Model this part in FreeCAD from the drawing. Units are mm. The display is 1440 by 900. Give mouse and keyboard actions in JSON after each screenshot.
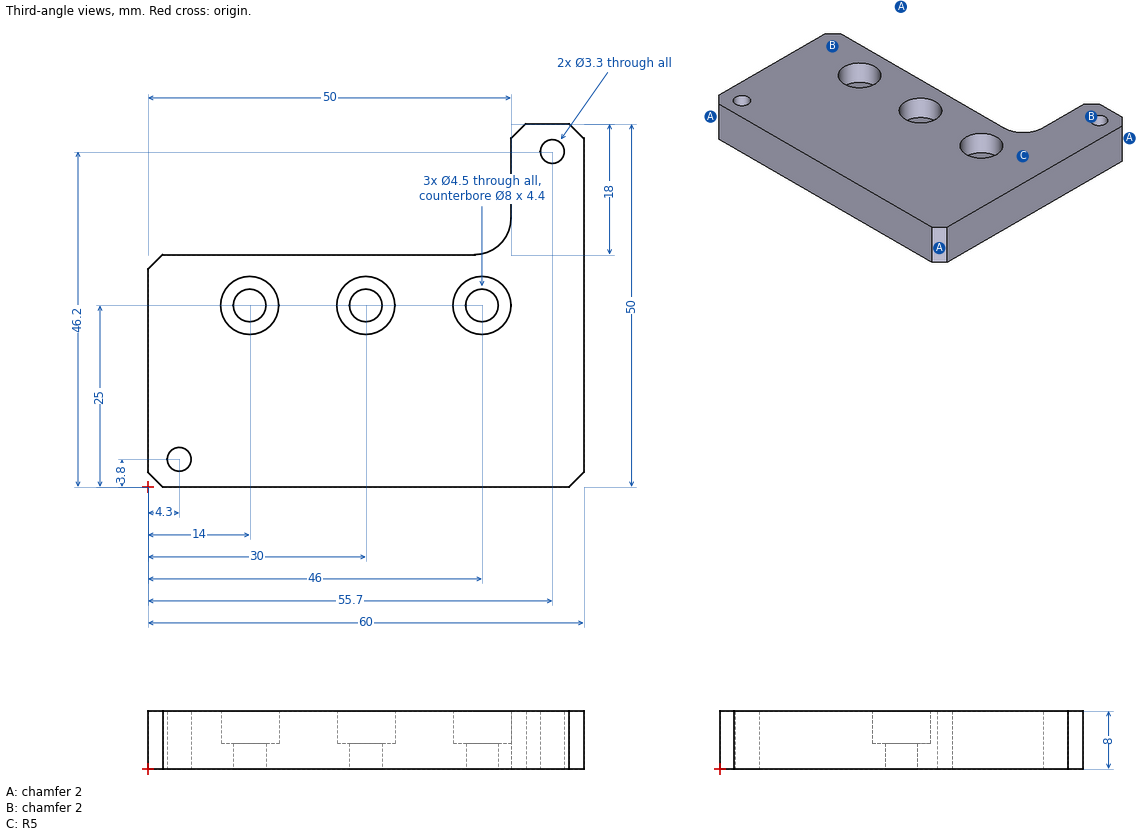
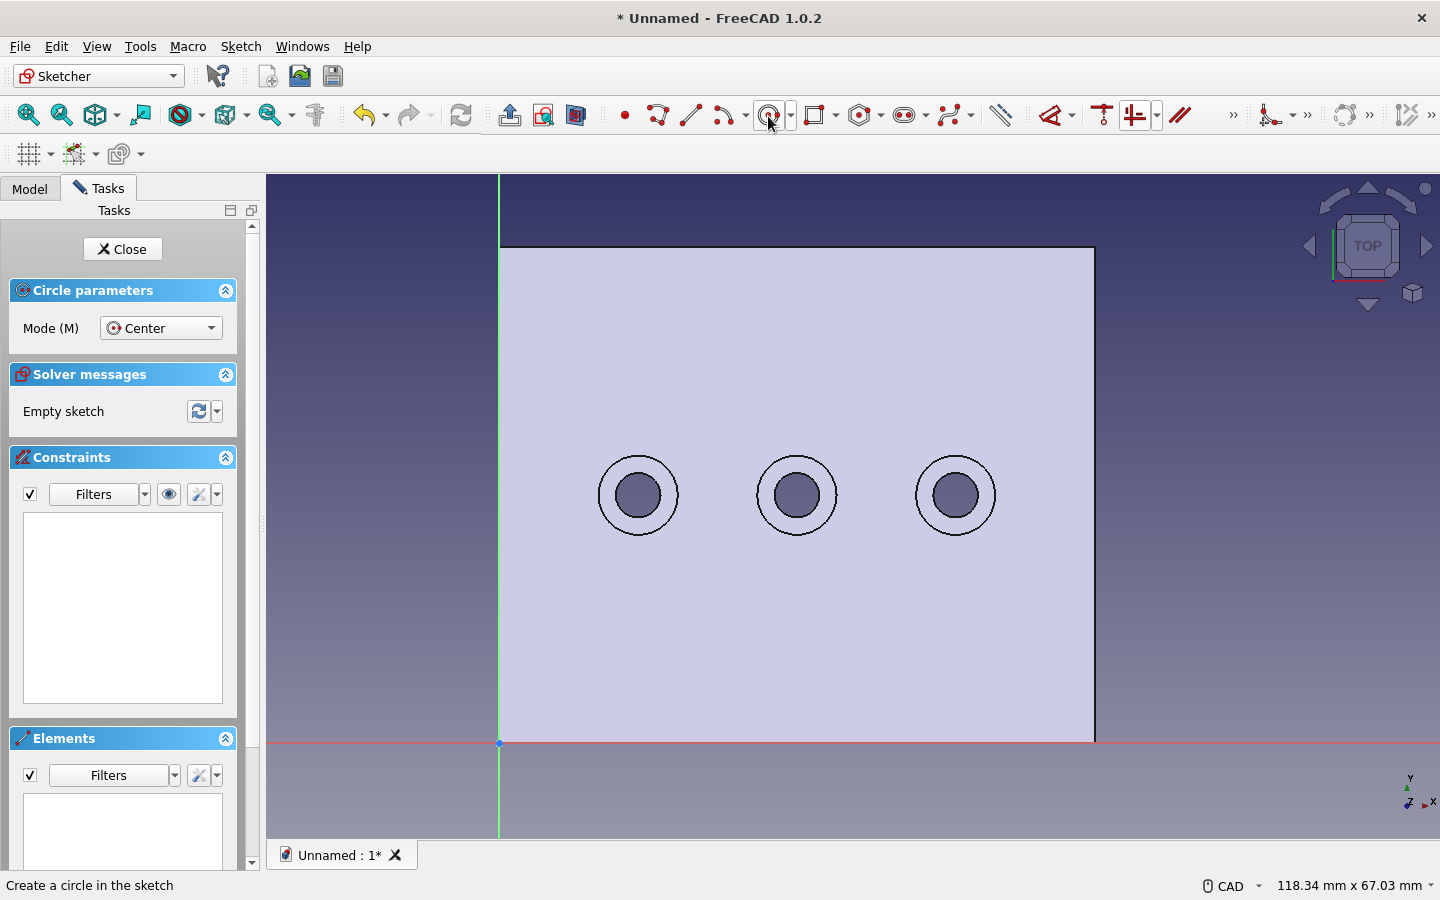
{"action": "scroll", "coordinate": [1052, 285], "scroll_direction": "up", "scroll_amount": 2}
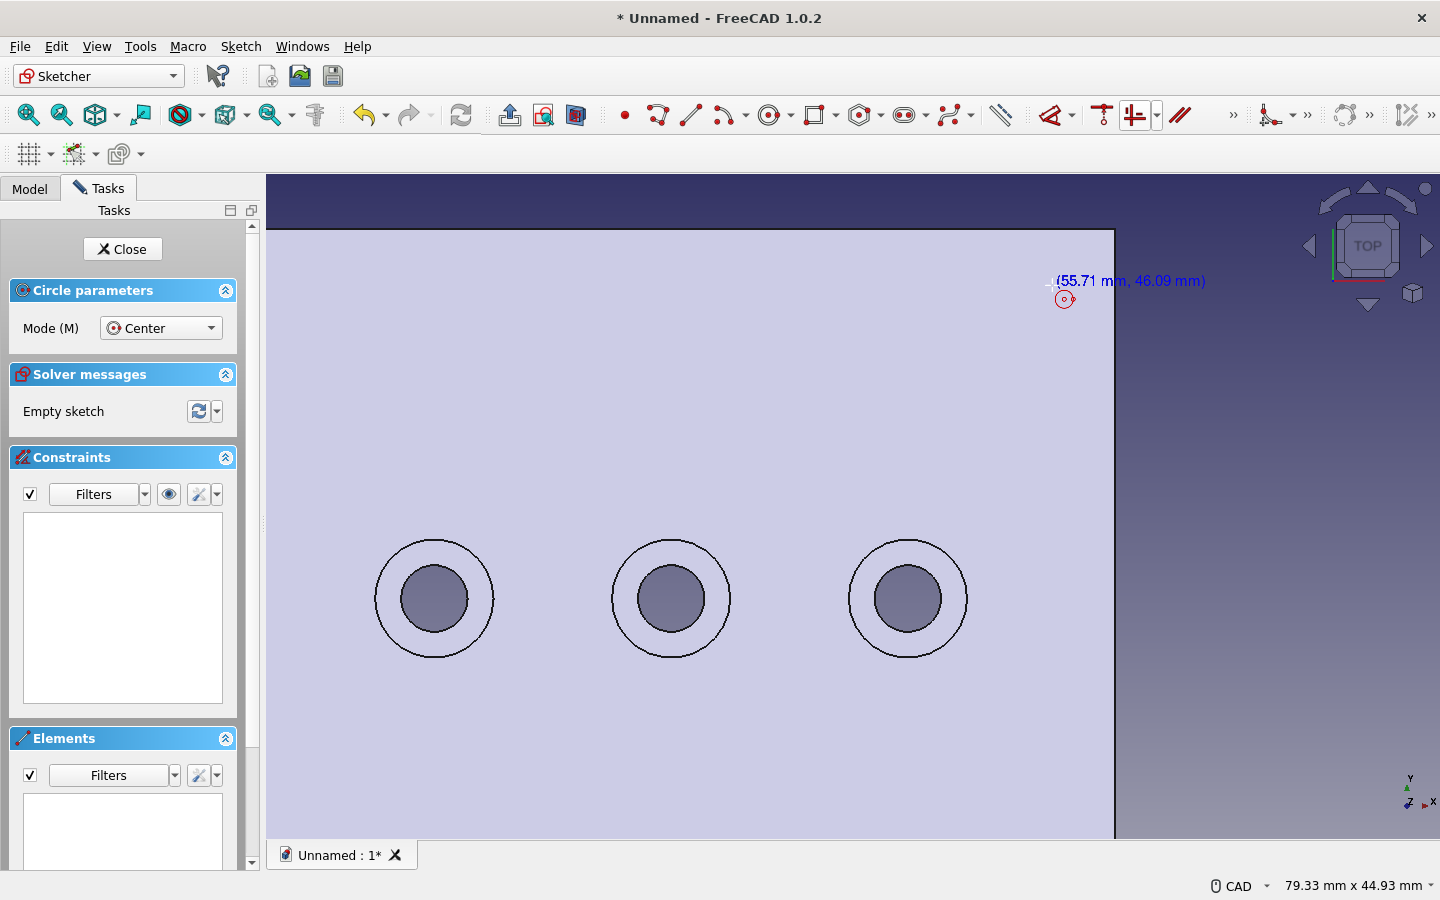
{"action": "left_click", "coordinate": [1051, 285]}
{"action": "mouse_move", "coordinate": [1069, 268]}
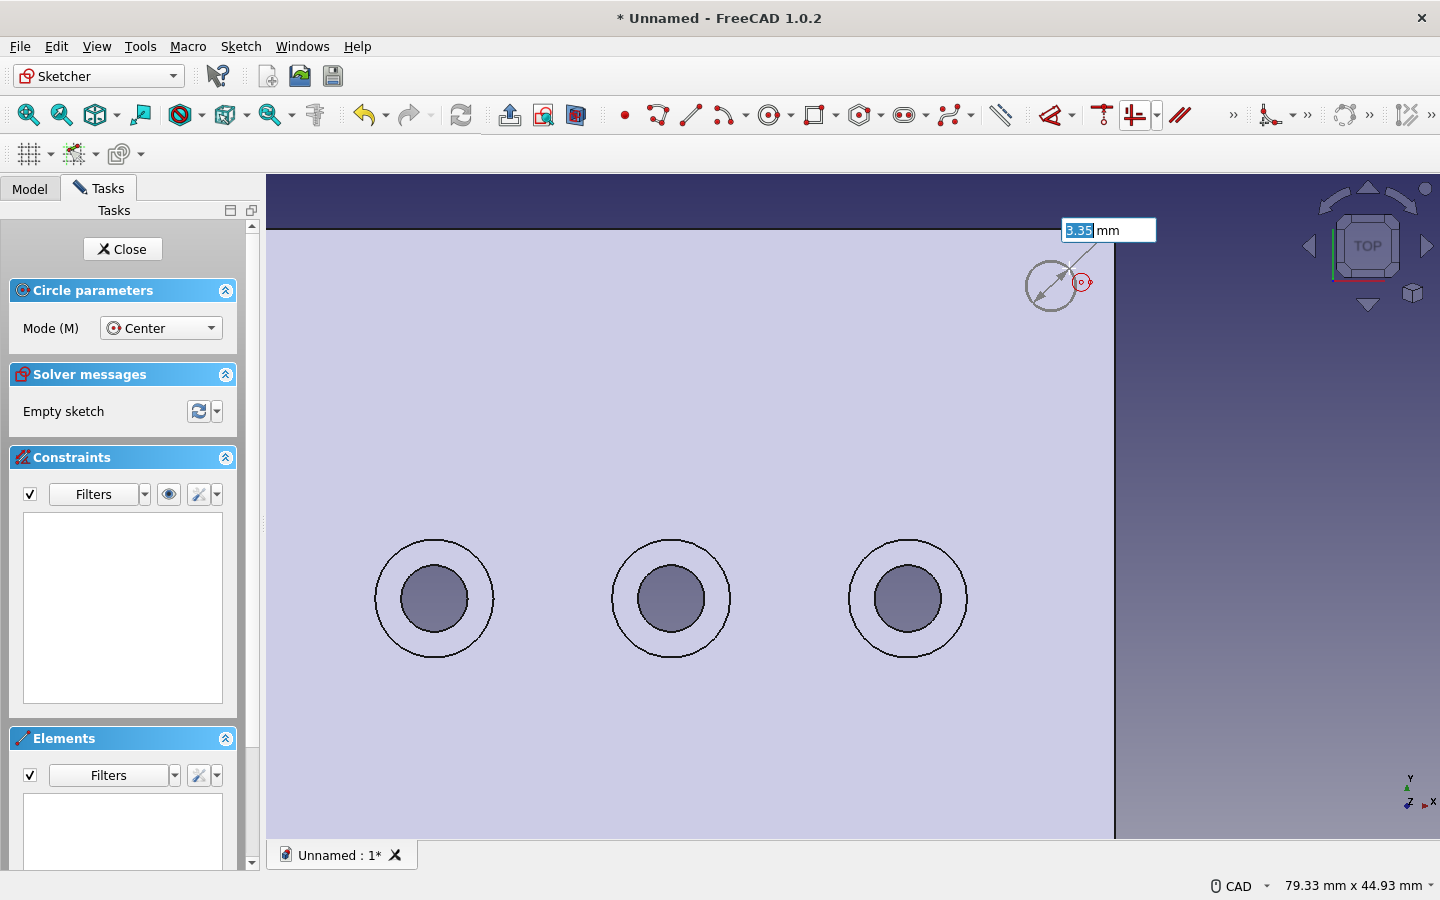
{"action": "type", "text": "3.3"}
{"action": "key", "text": "Return"}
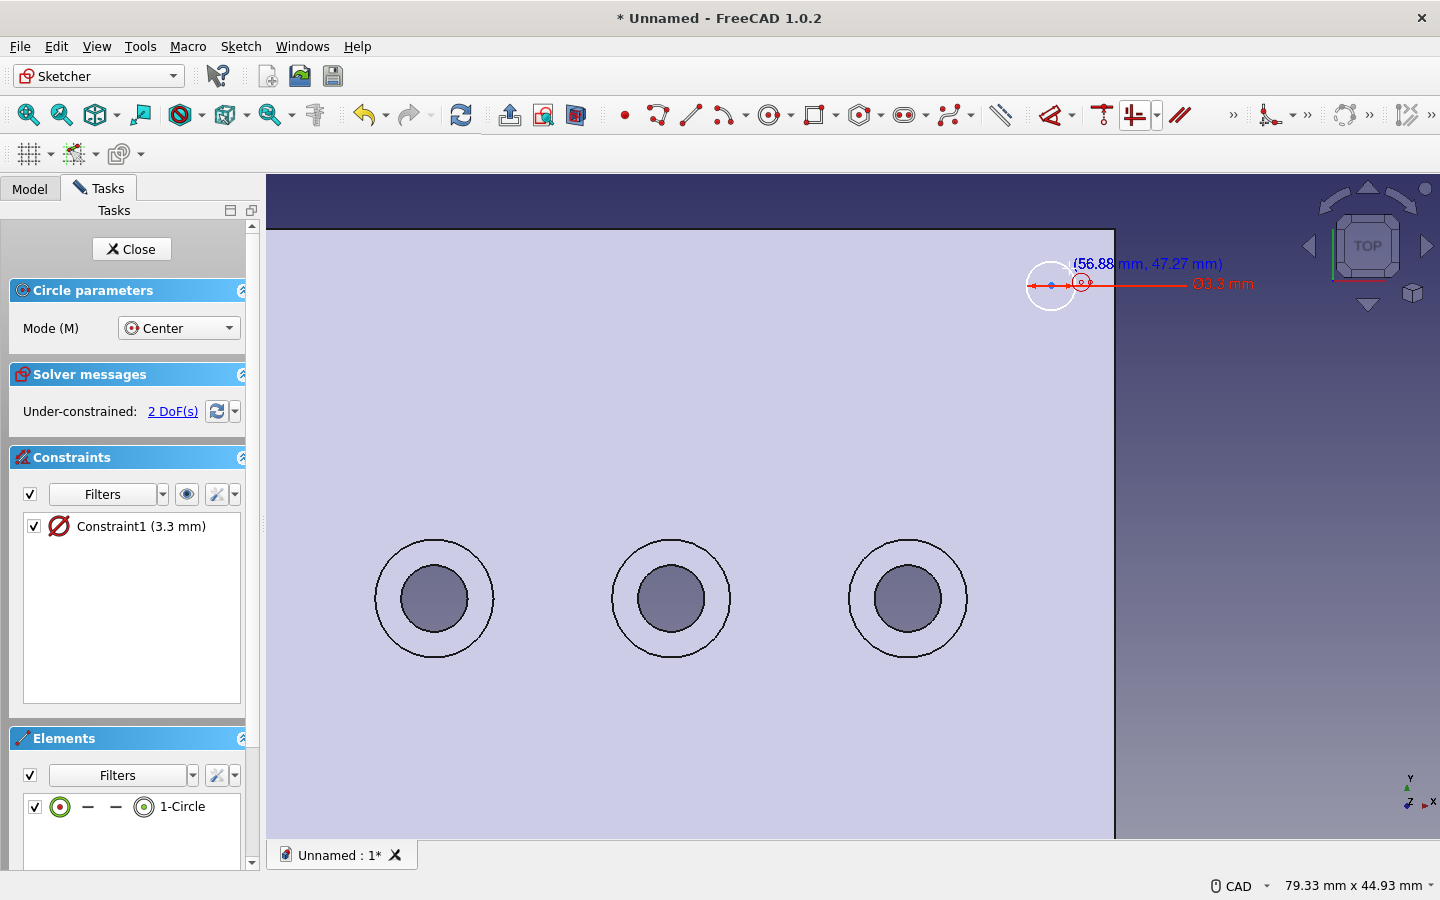
{"action": "scroll", "coordinate": [1055, 287], "scroll_direction": "down", "scroll_amount": 2}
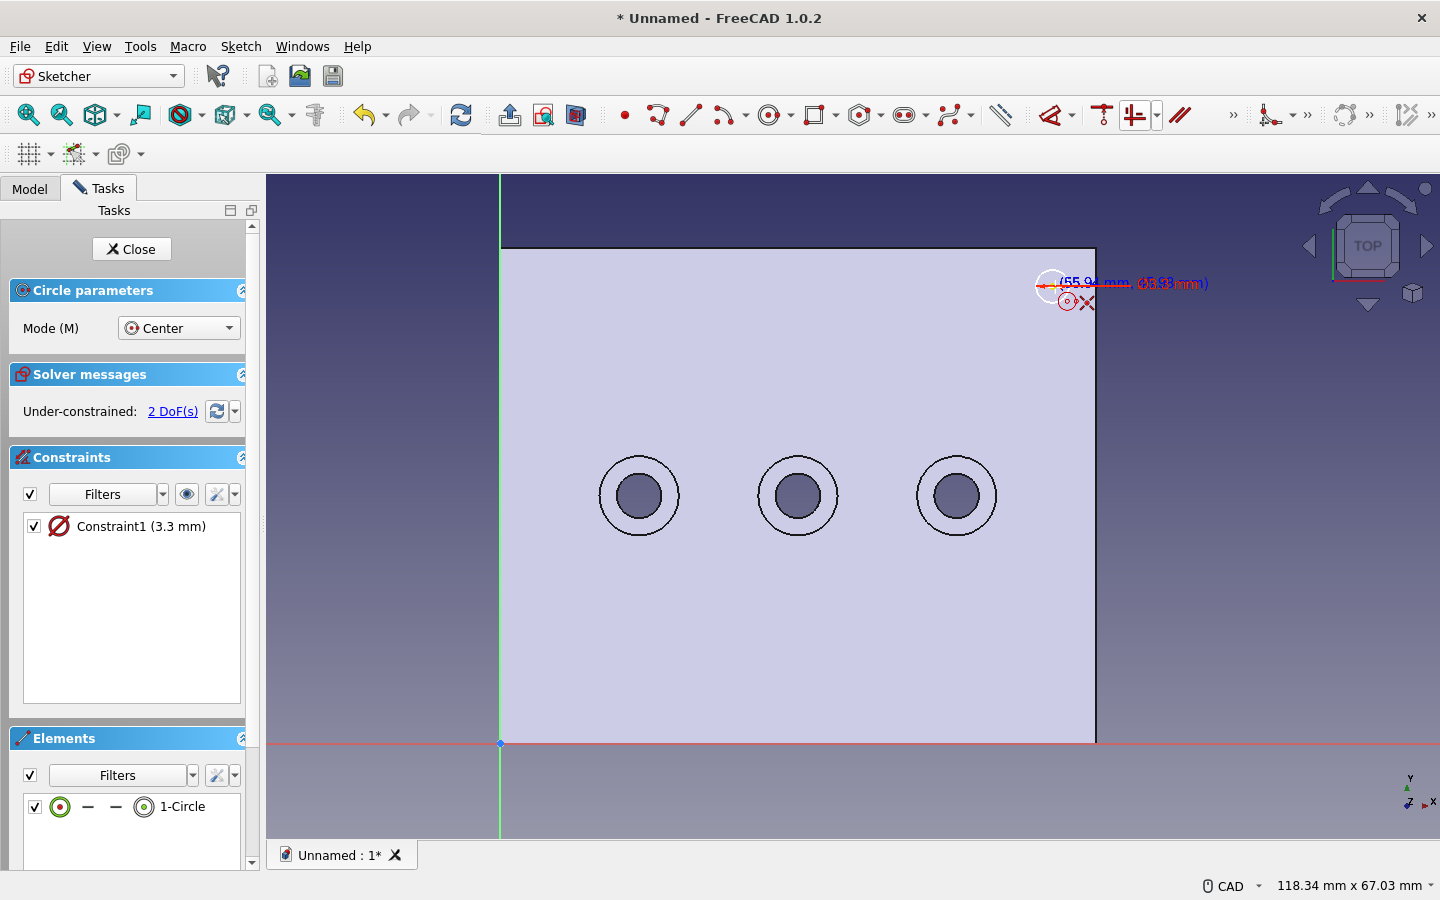
{"action": "scroll", "coordinate": [543, 706], "scroll_direction": "up", "scroll_amount": 2}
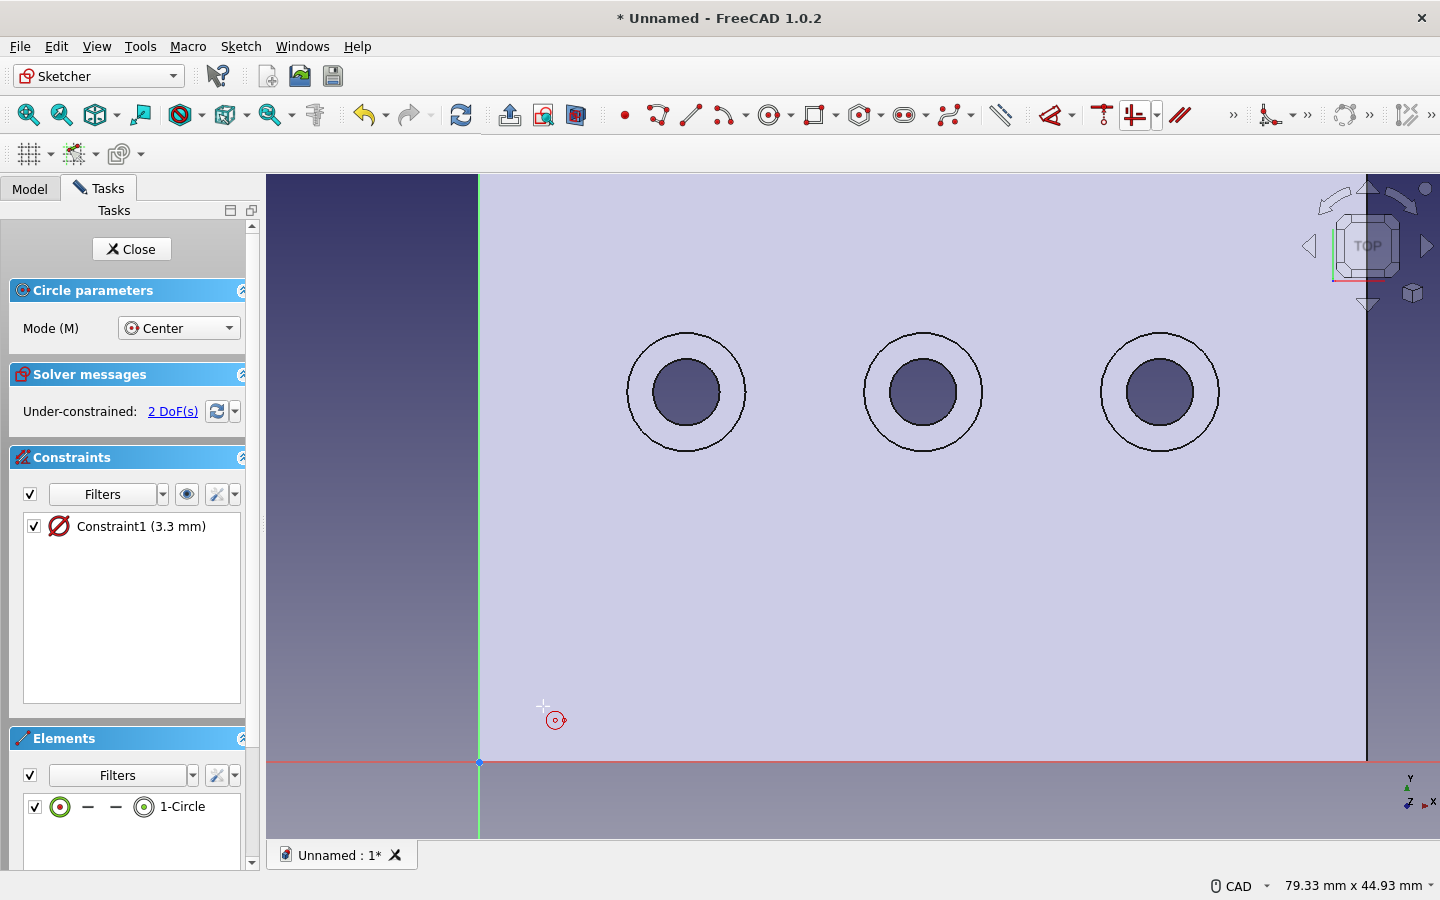
{"action": "left_click", "coordinate": [543, 706]}
{"action": "mouse_move", "coordinate": [560, 689]}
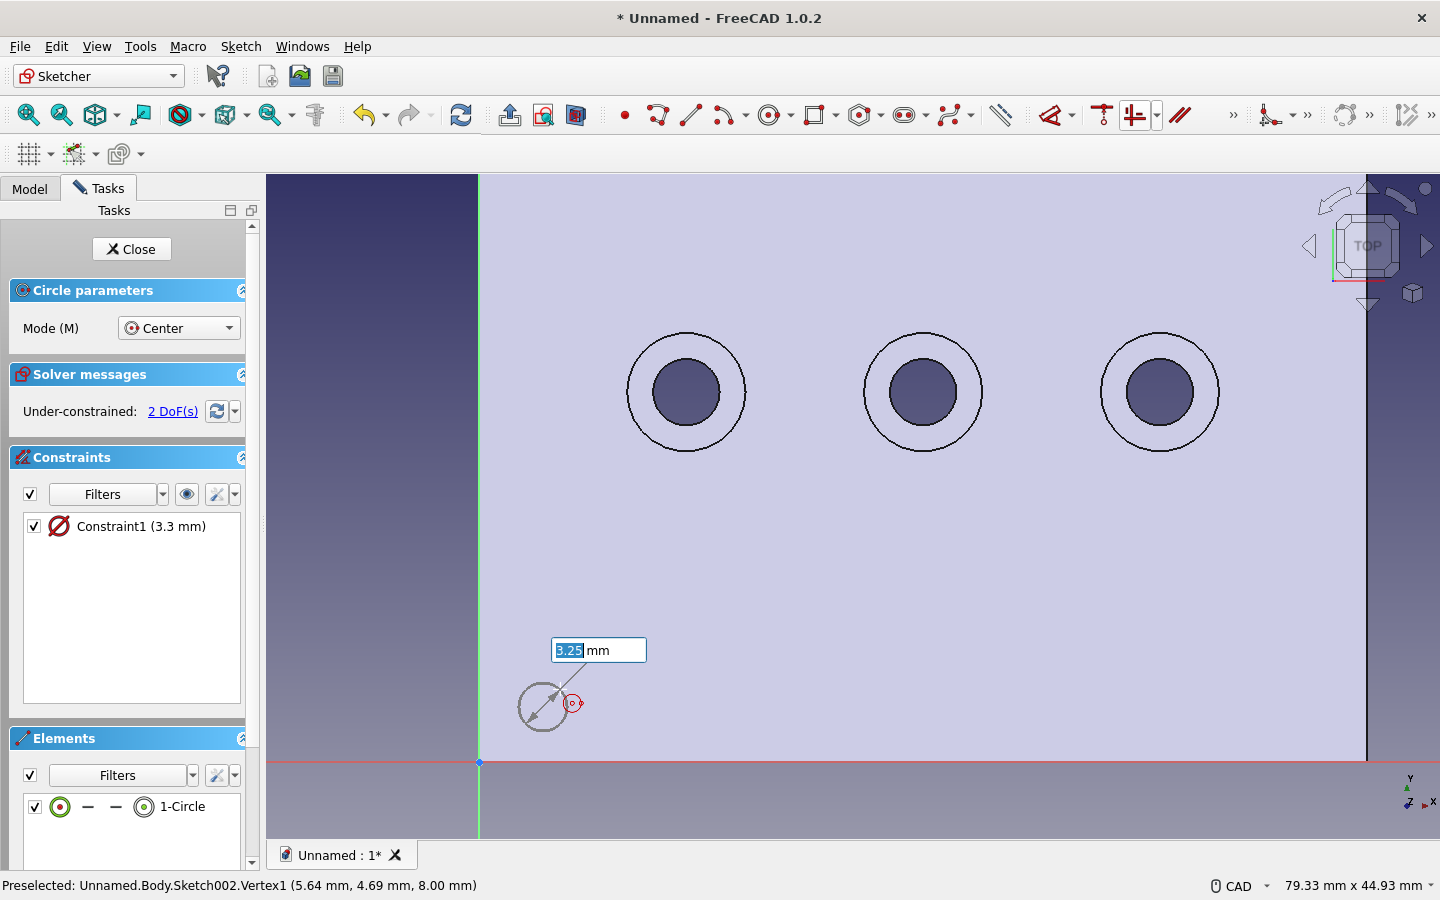
{"action": "type", "text": "3.3"}
{"action": "key", "text": "Return"}
{"action": "key", "text": "Escape"}